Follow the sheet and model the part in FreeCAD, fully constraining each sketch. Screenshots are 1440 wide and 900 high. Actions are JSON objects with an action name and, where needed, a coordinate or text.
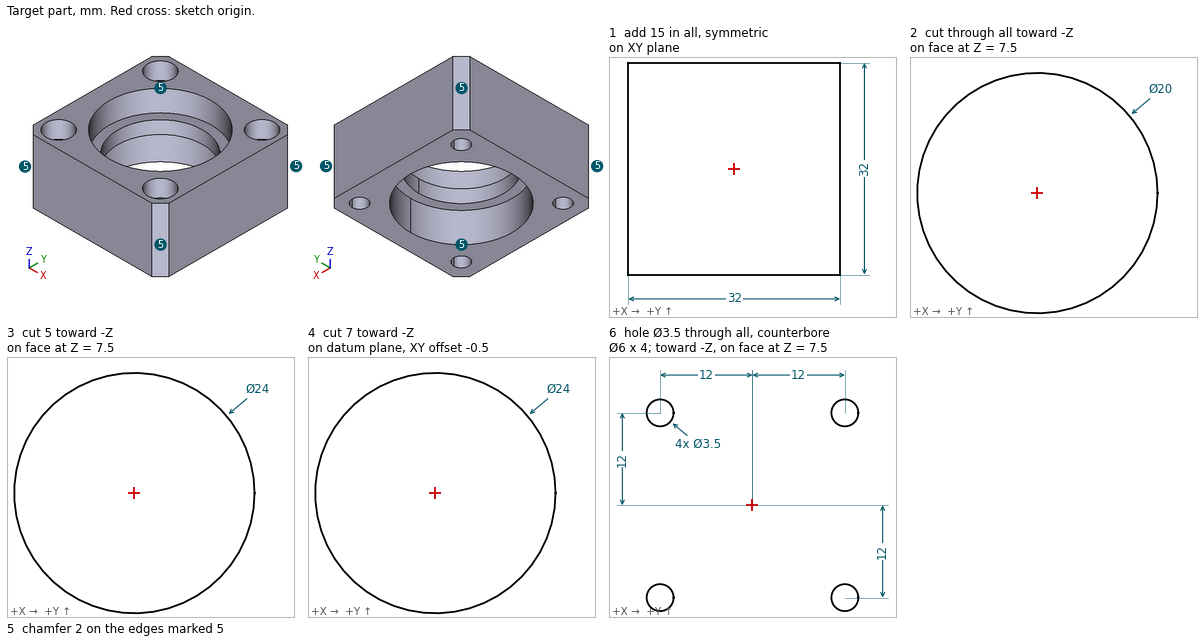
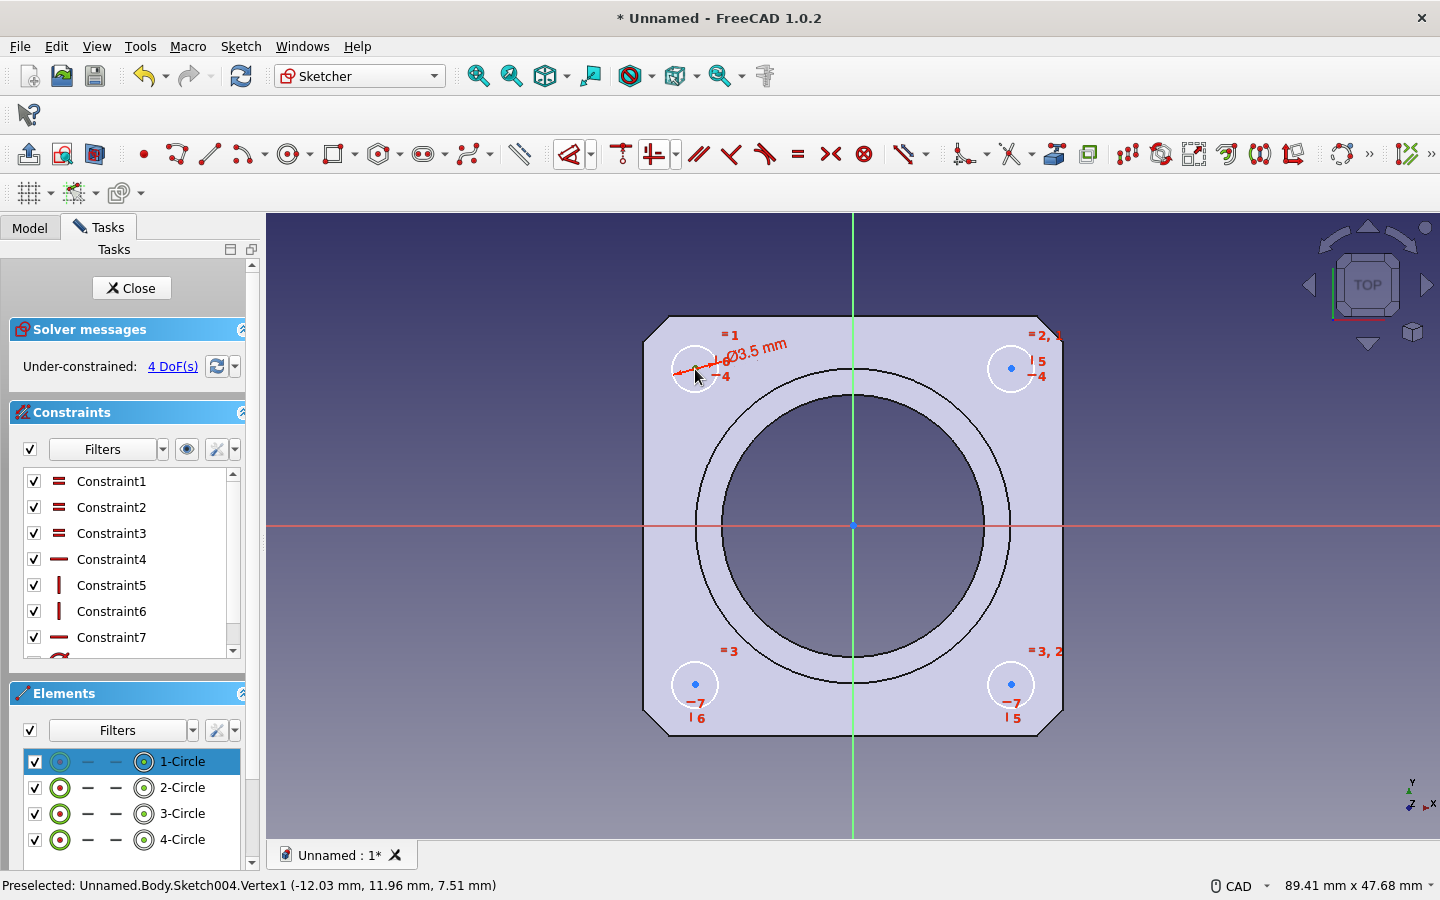
{"action": "left_click", "coordinate": [590, 154]}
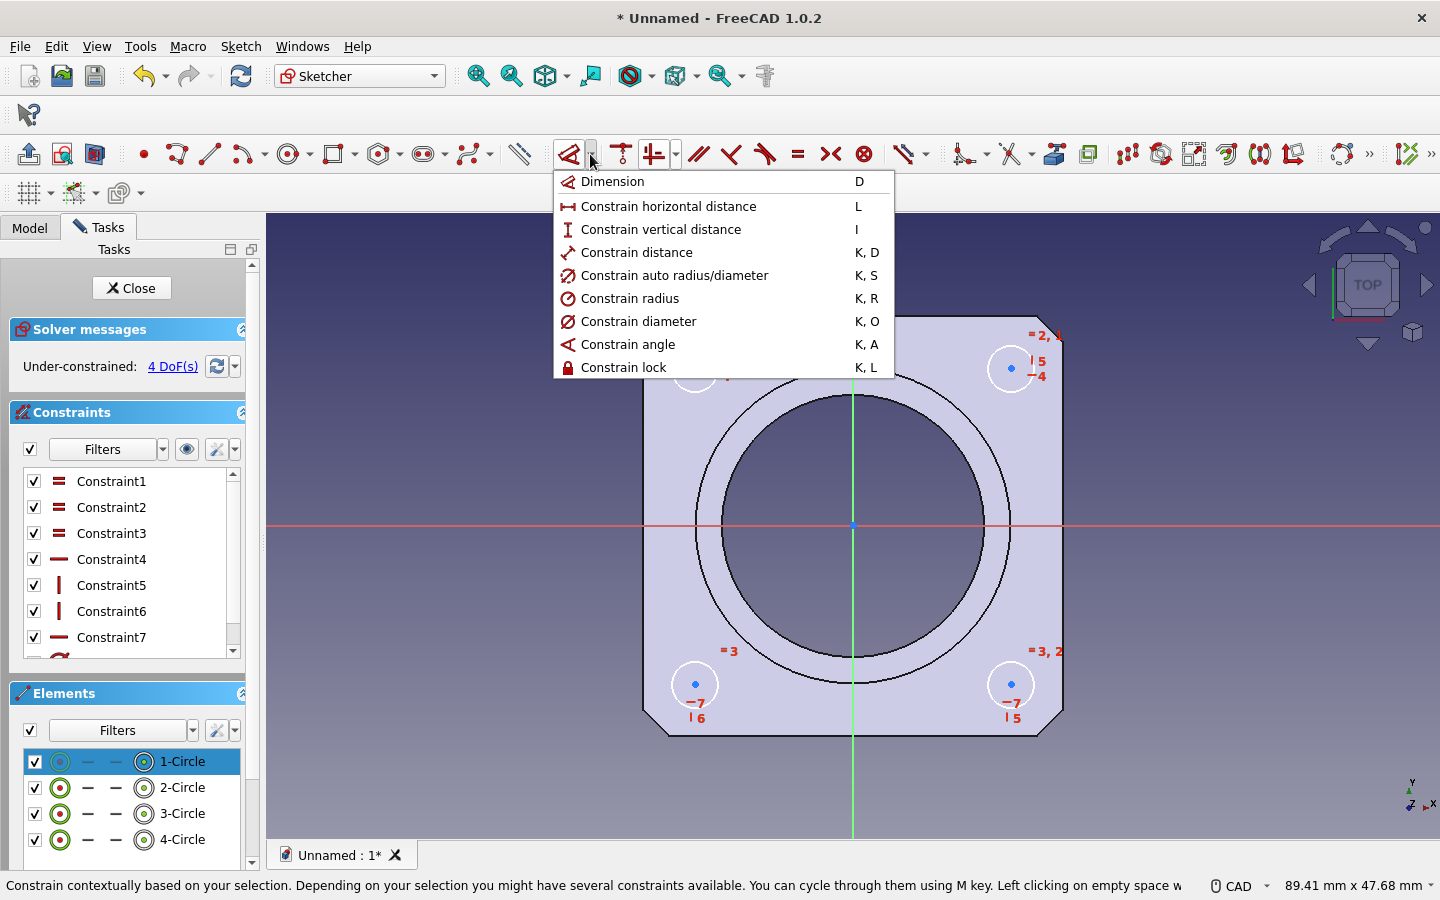
{"action": "left_click", "coordinate": [724, 206]}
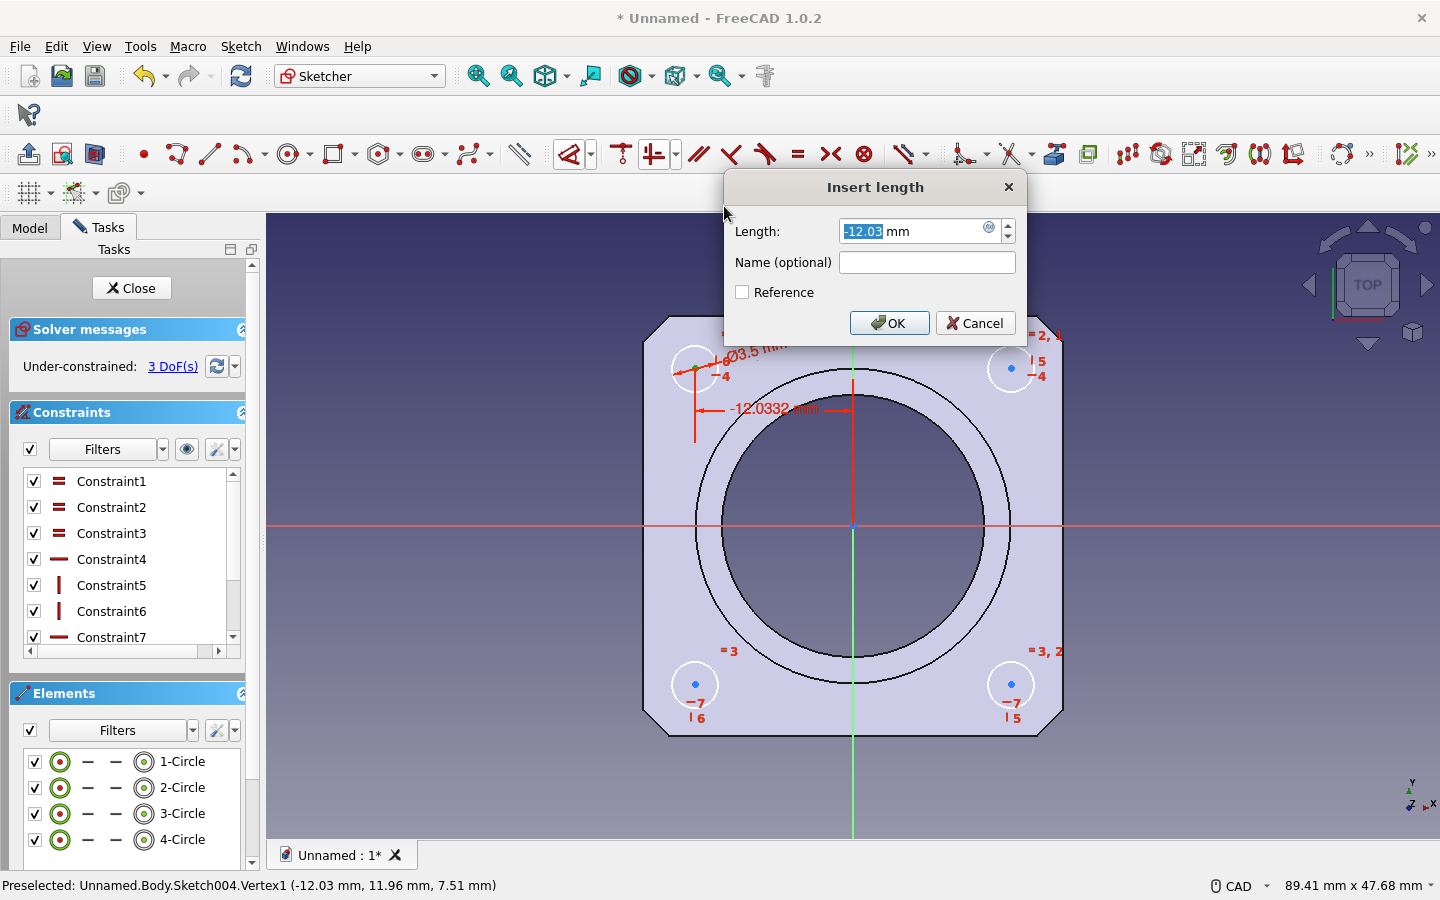
{"action": "type", "text": "-12"}
{"action": "key", "text": "Return"}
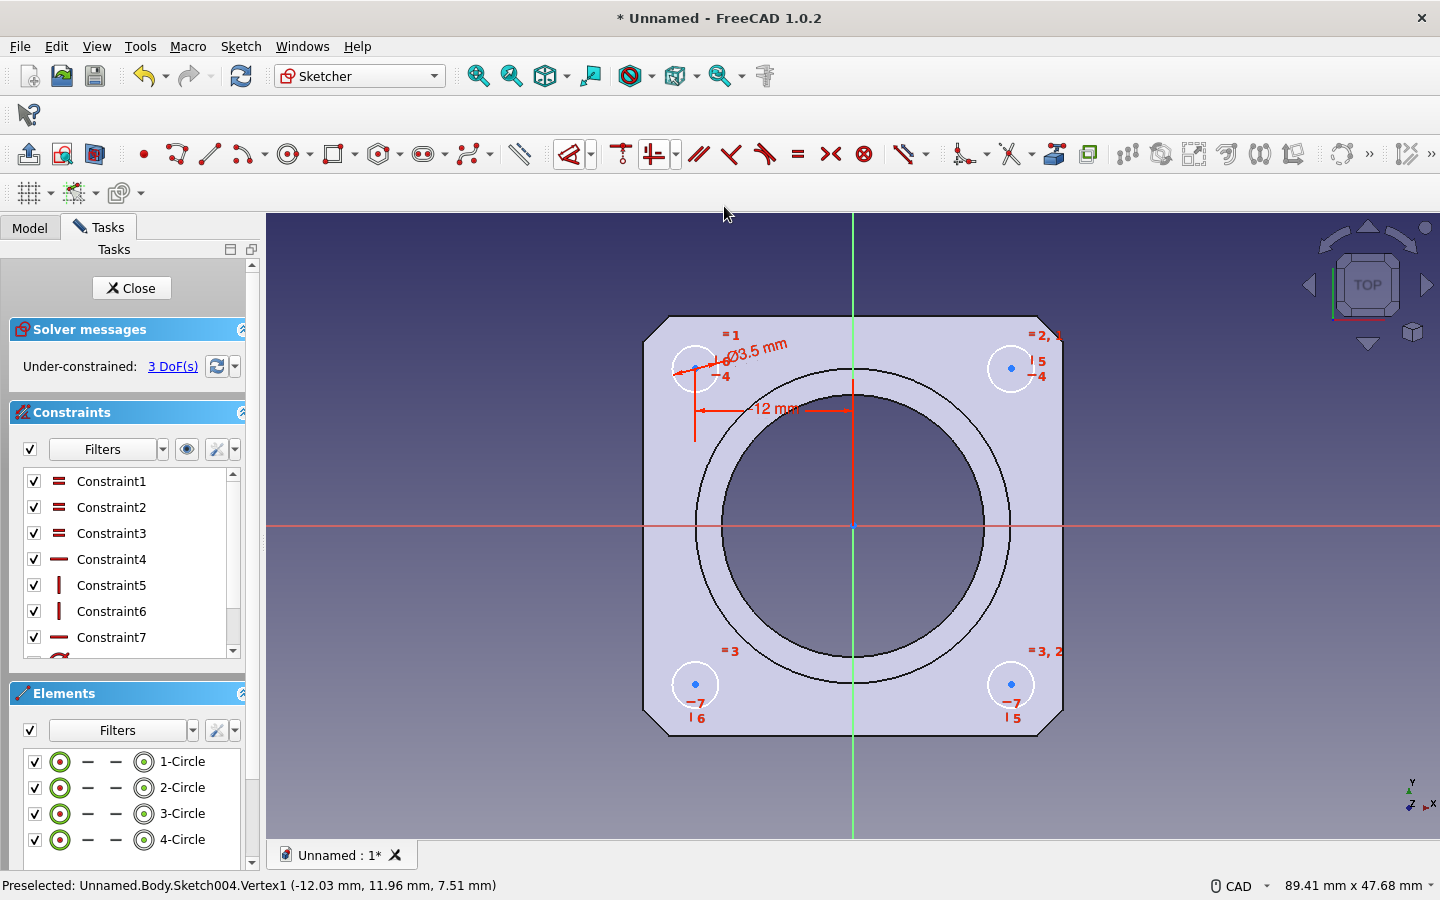
{"action": "left_click", "coordinate": [695, 369]}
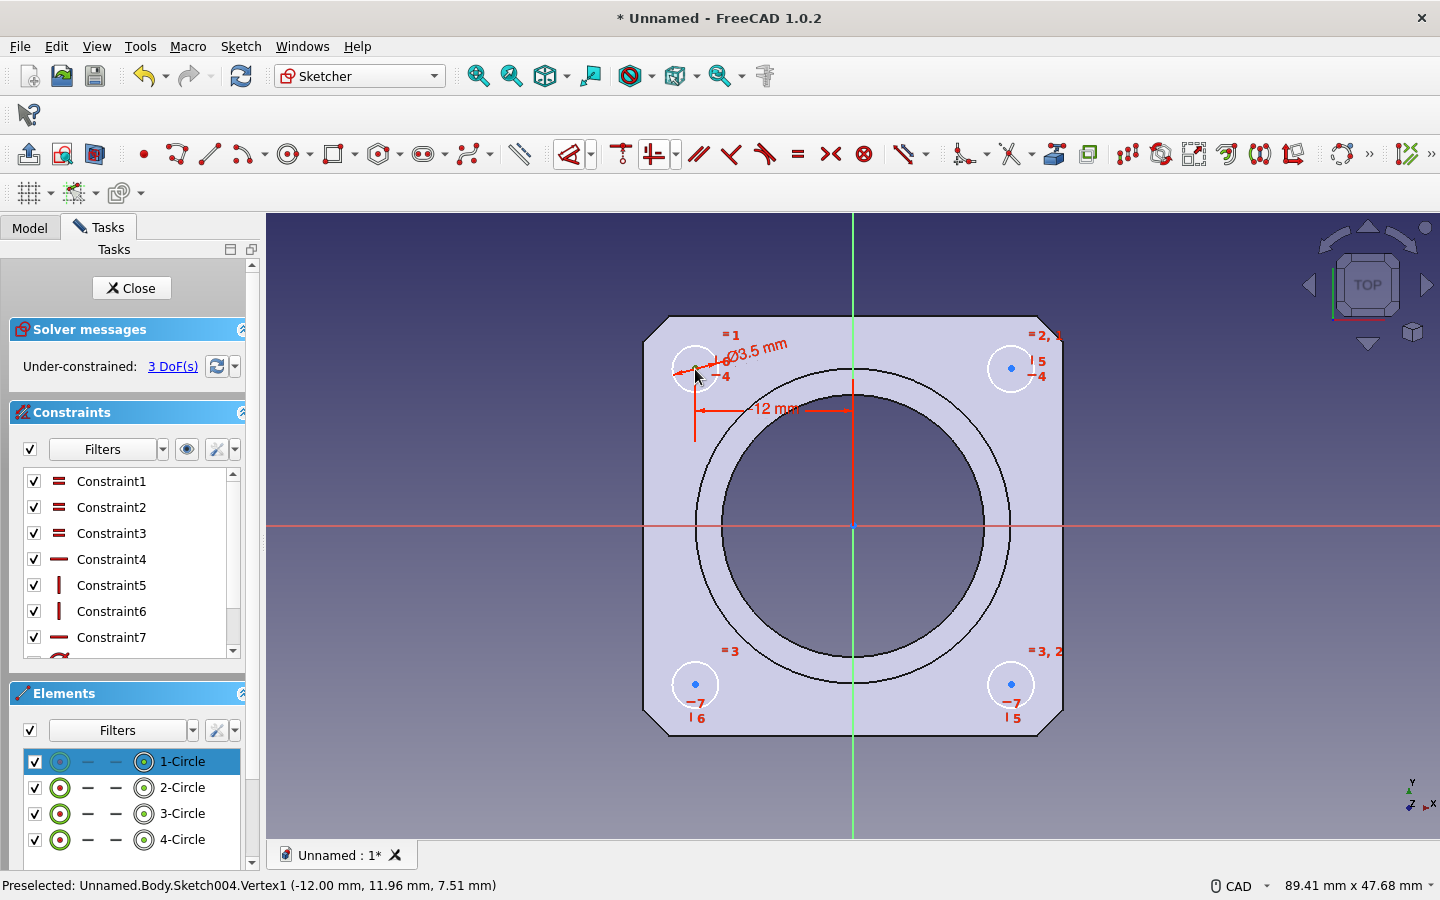
{"action": "left_click", "coordinate": [590, 154]}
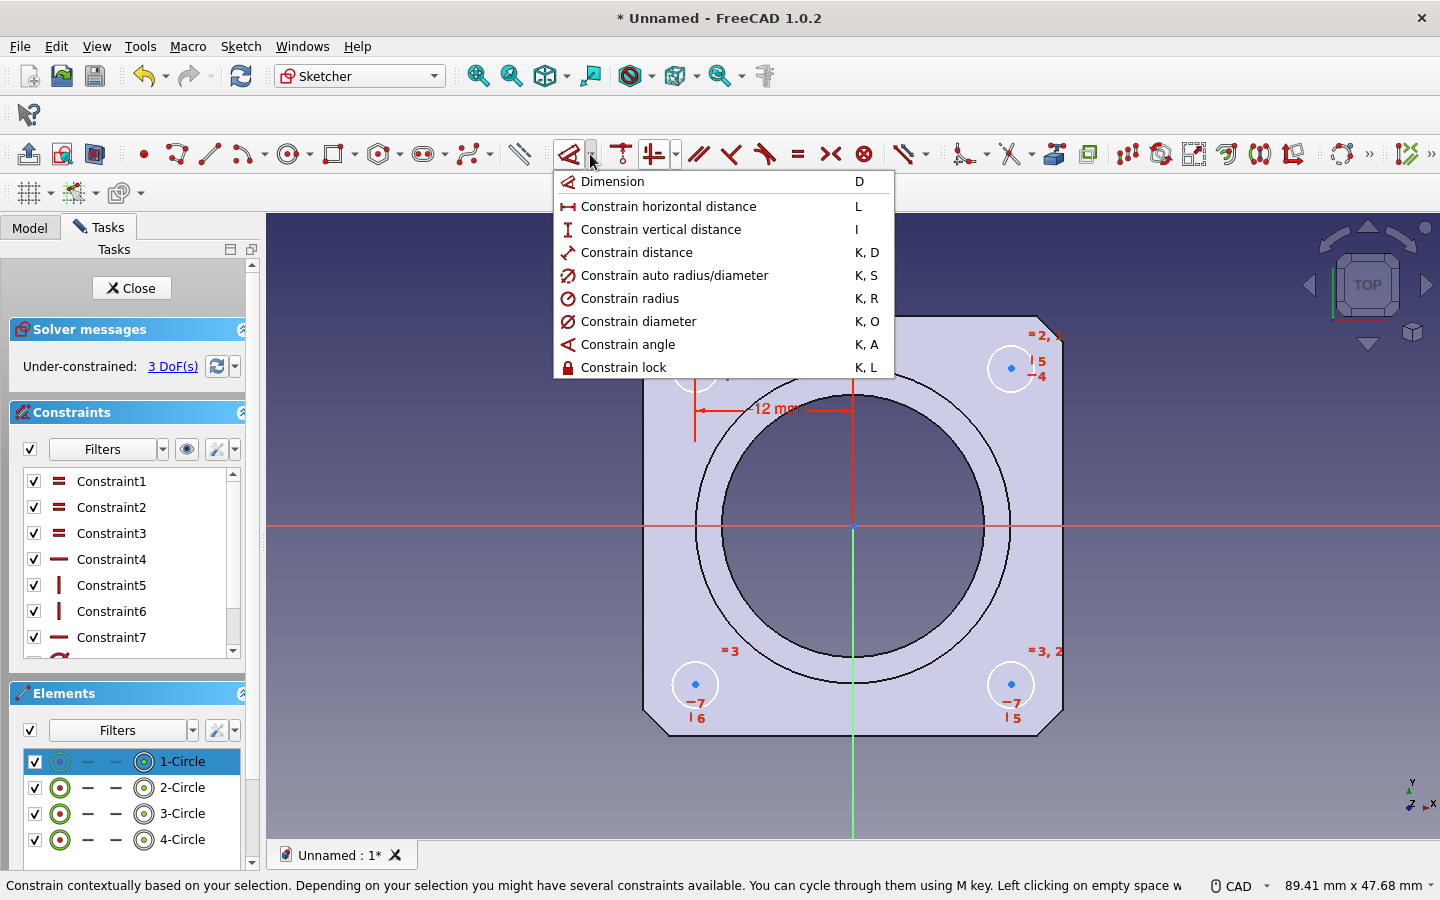
{"action": "left_click", "coordinate": [724, 230]}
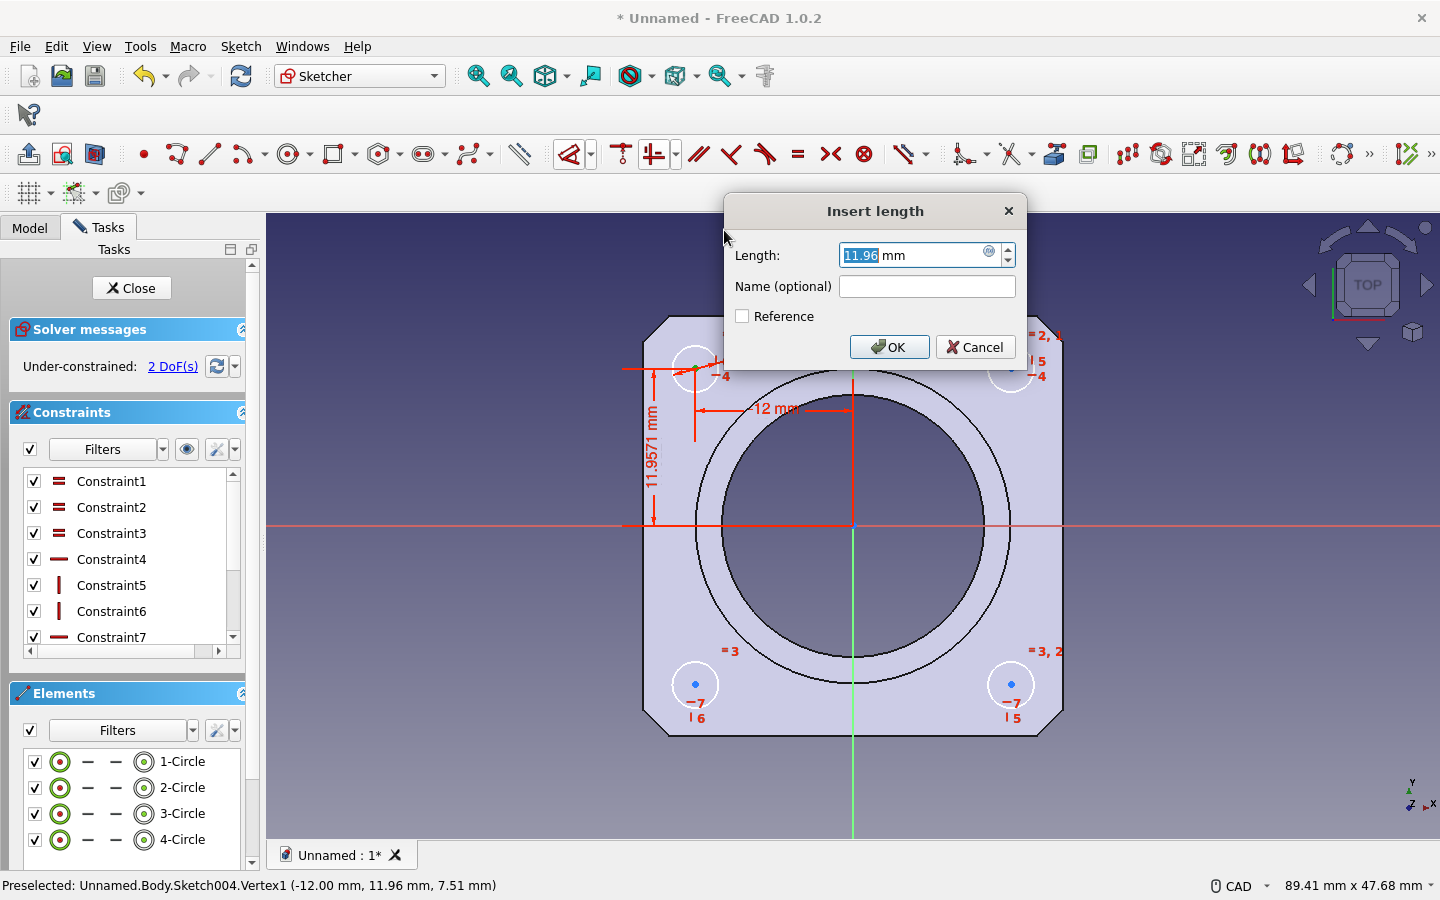
{"action": "type", "text": "12"}
{"action": "key", "text": "Return"}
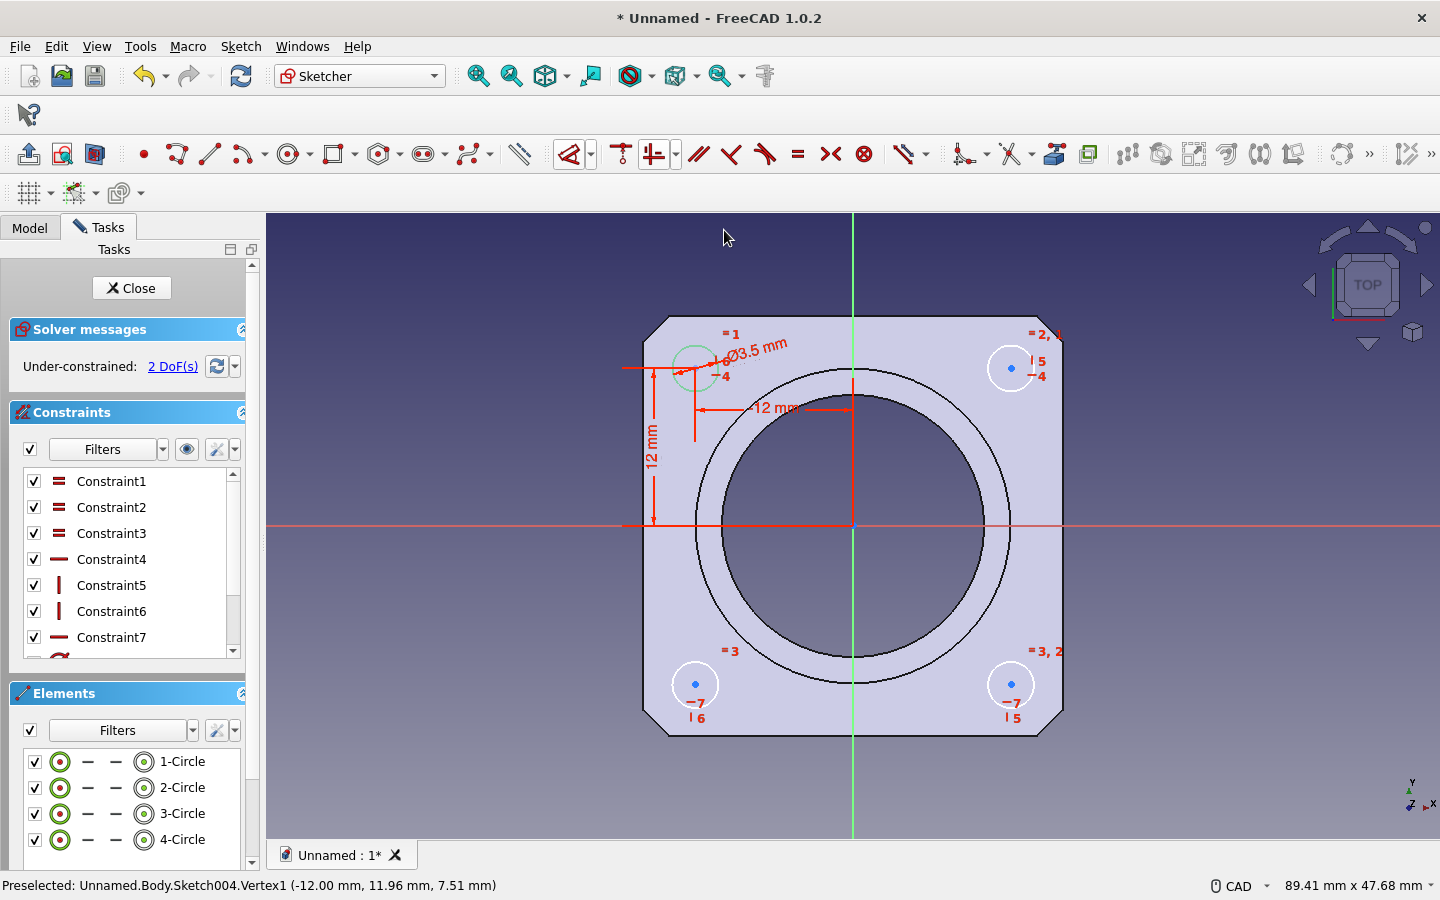
{"action": "left_click", "coordinate": [1011, 368]}